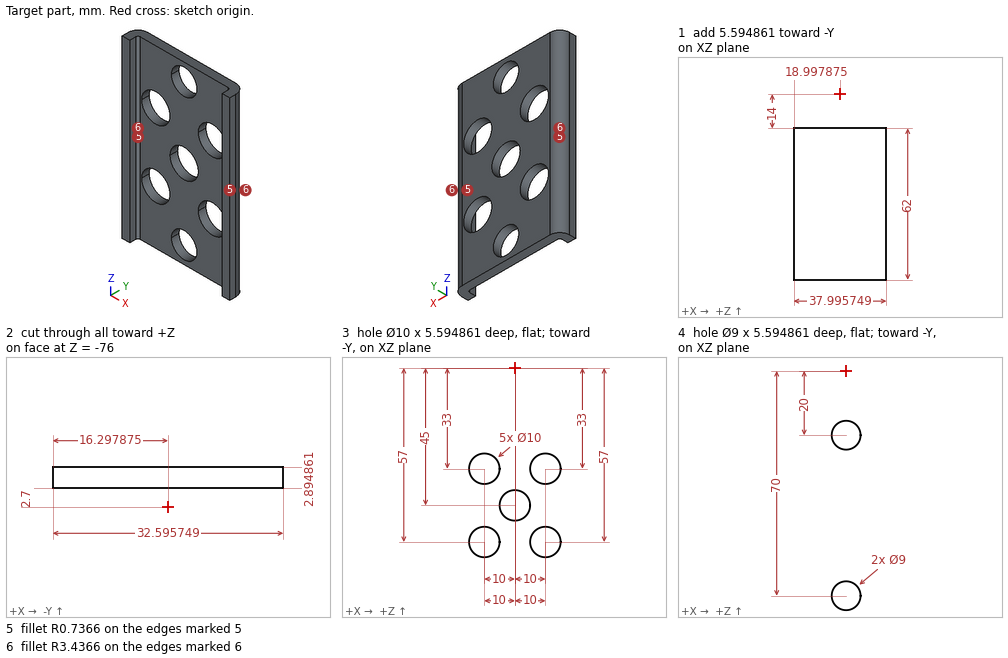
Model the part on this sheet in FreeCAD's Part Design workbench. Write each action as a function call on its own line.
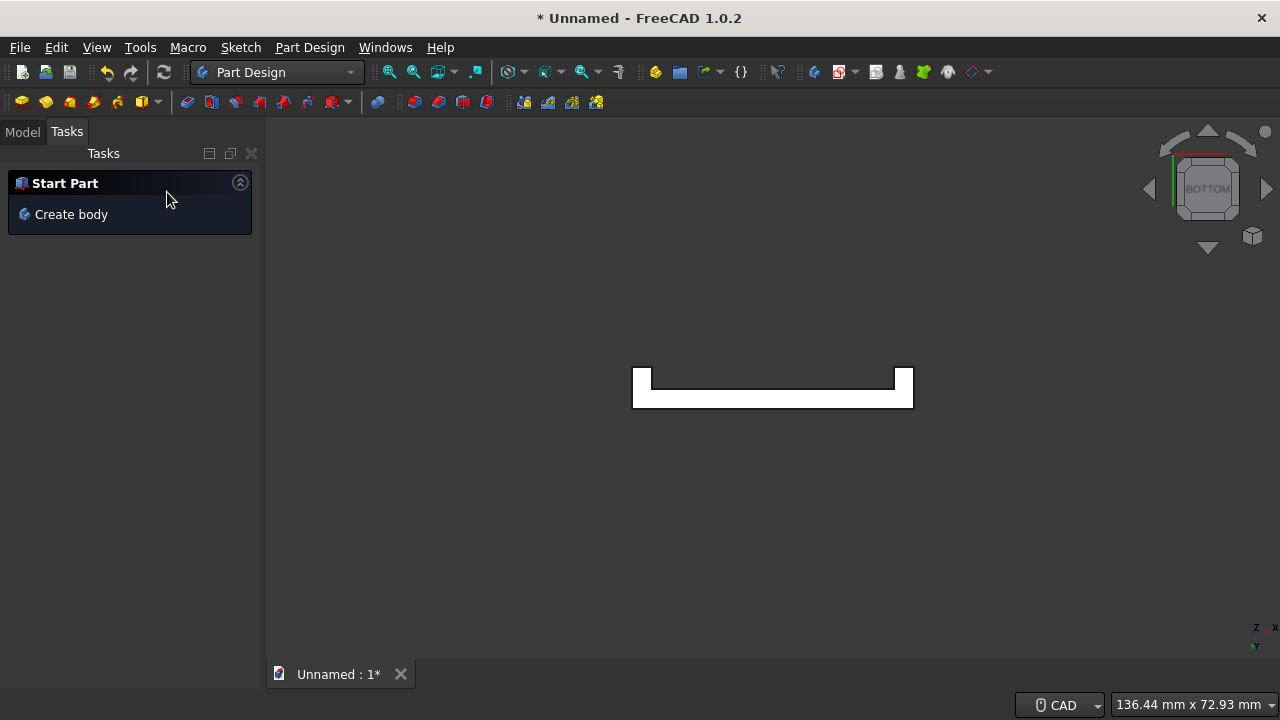
click(390, 72)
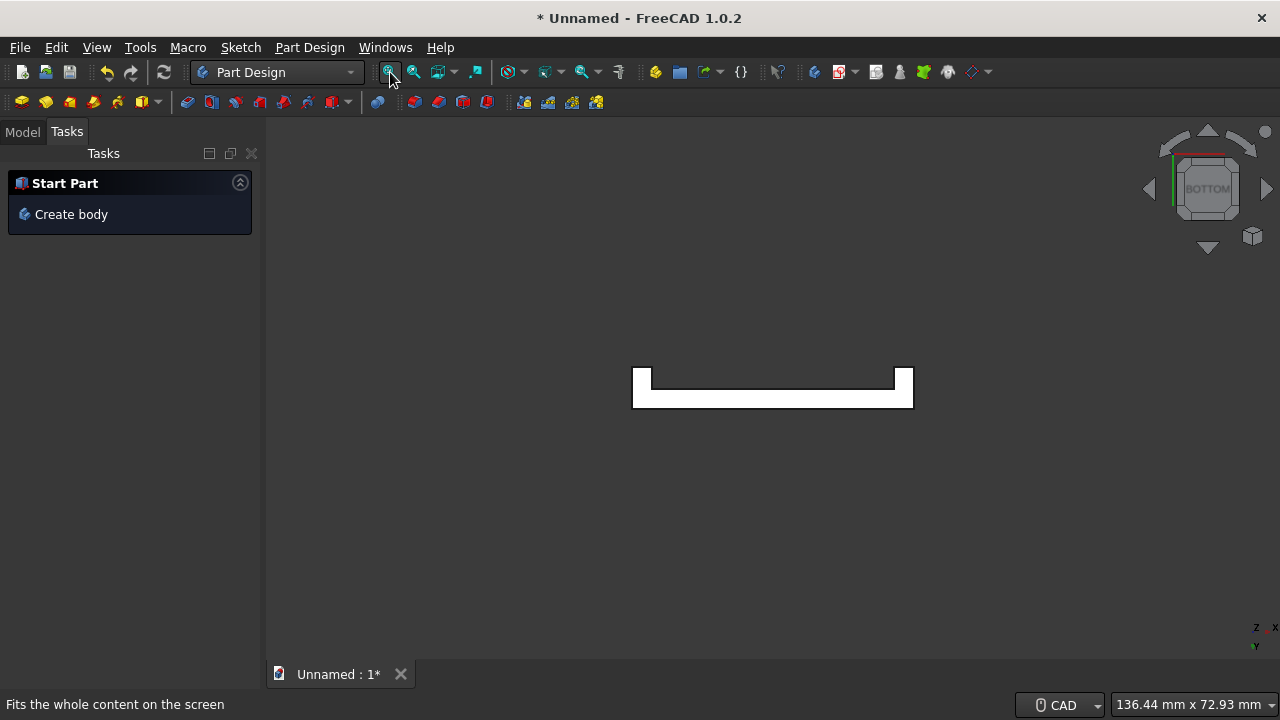
key(0)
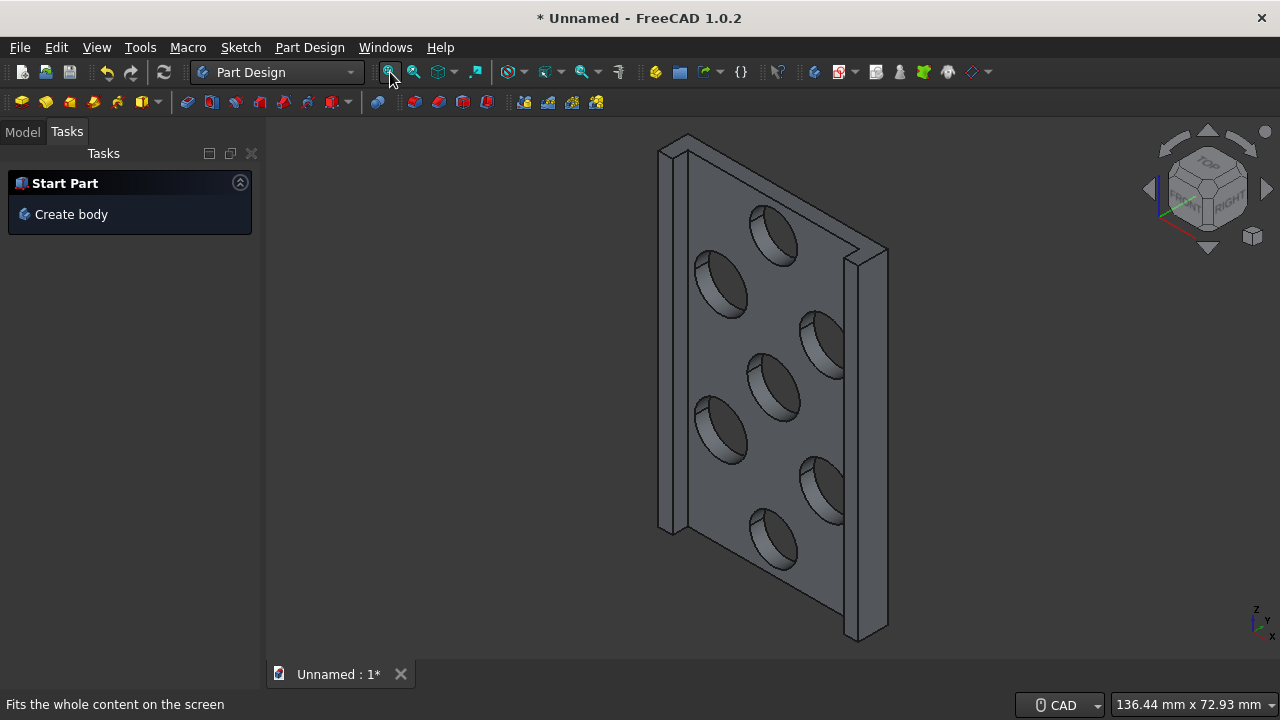
key(2)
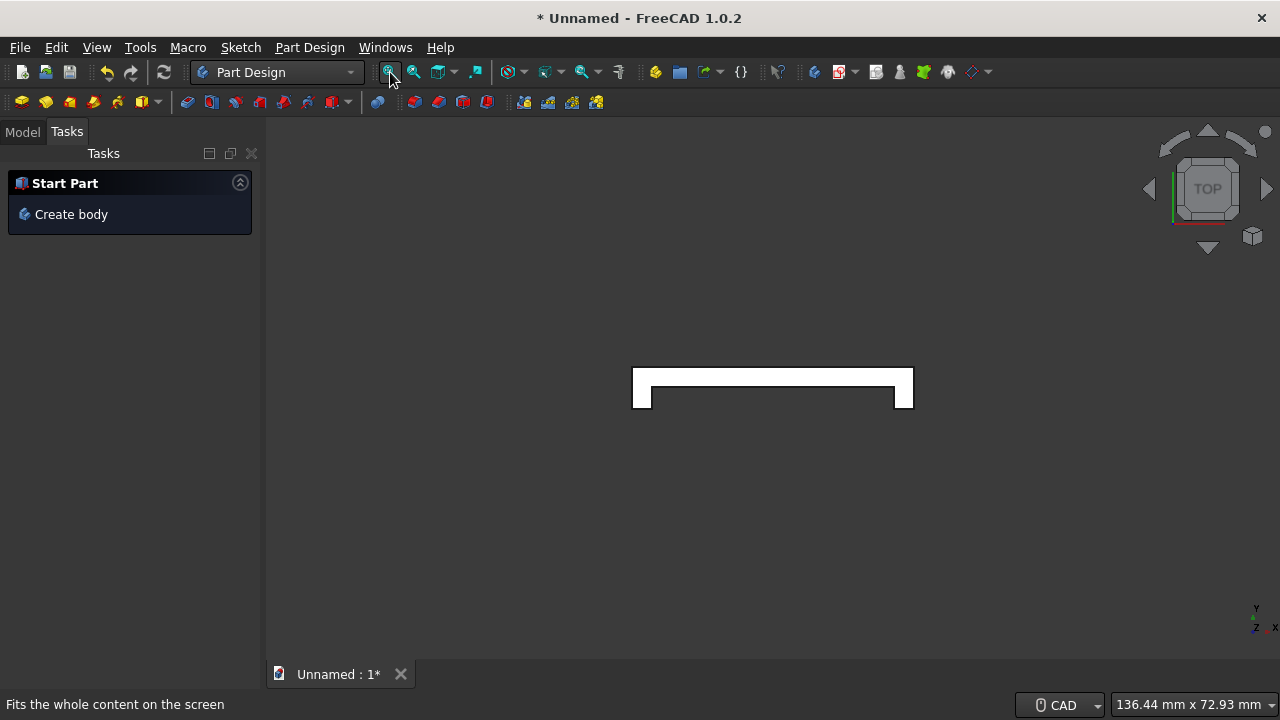
key(v)
key(f)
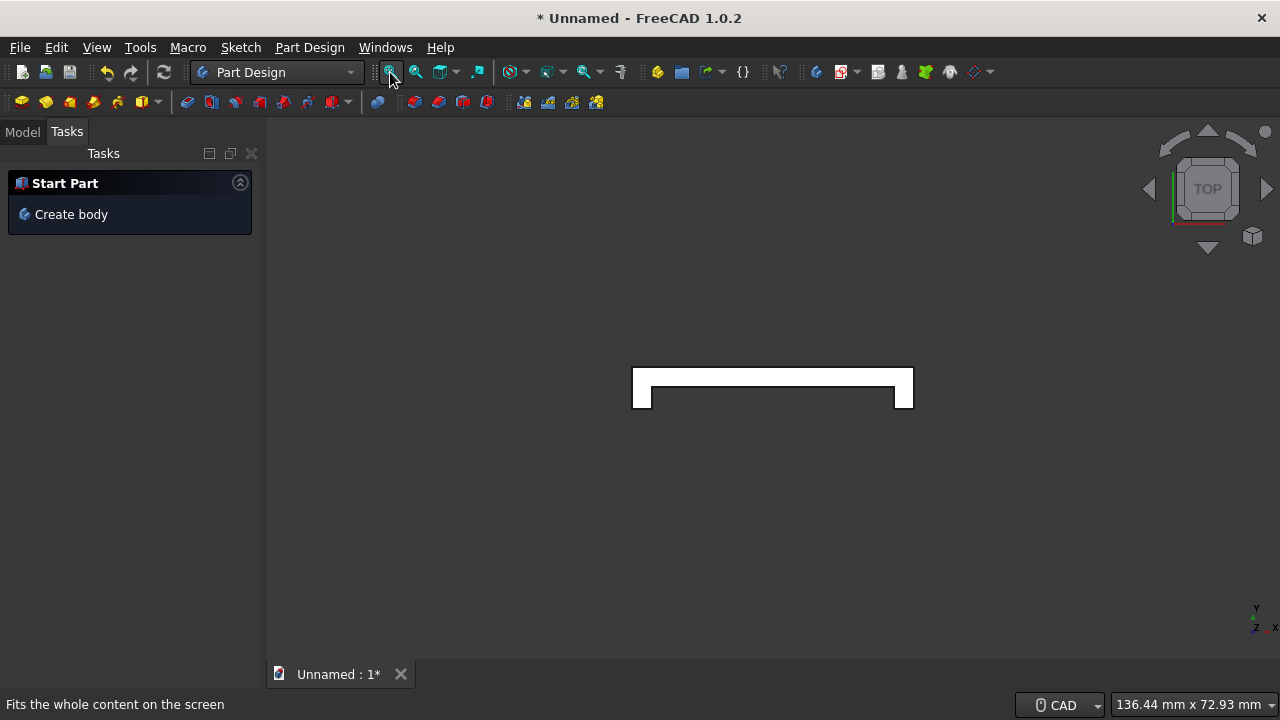
key(1)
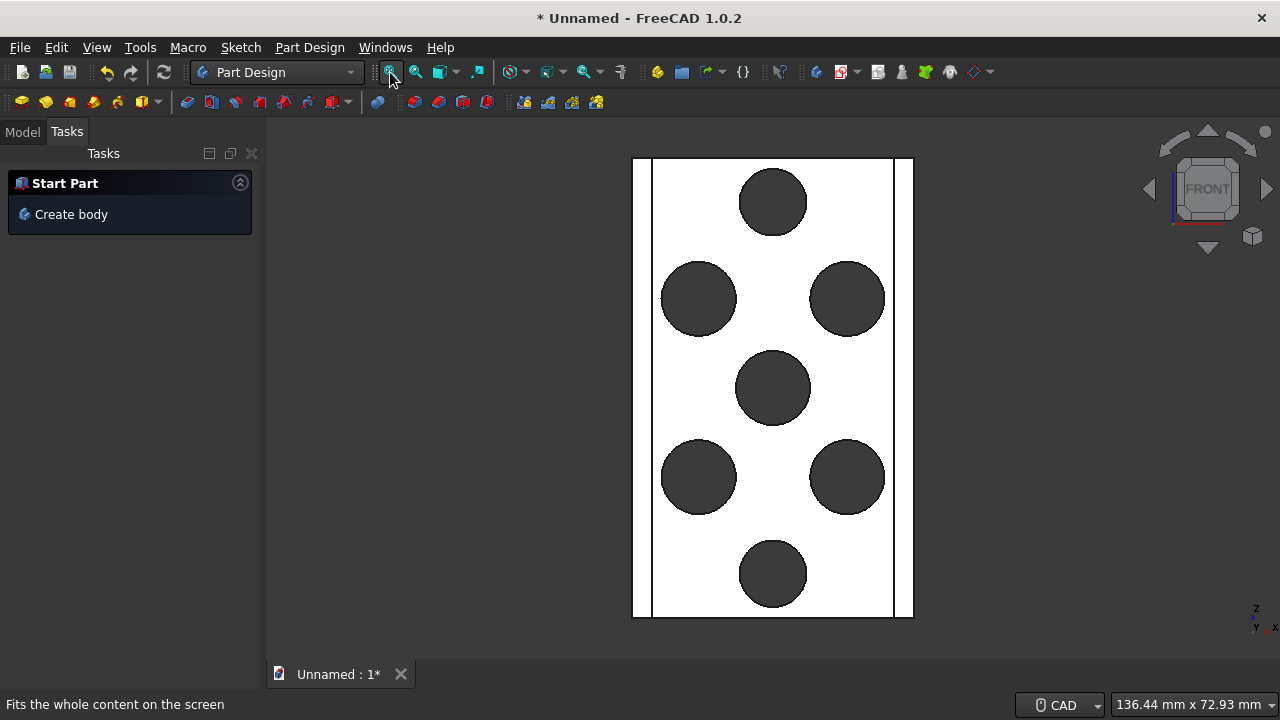
key(3)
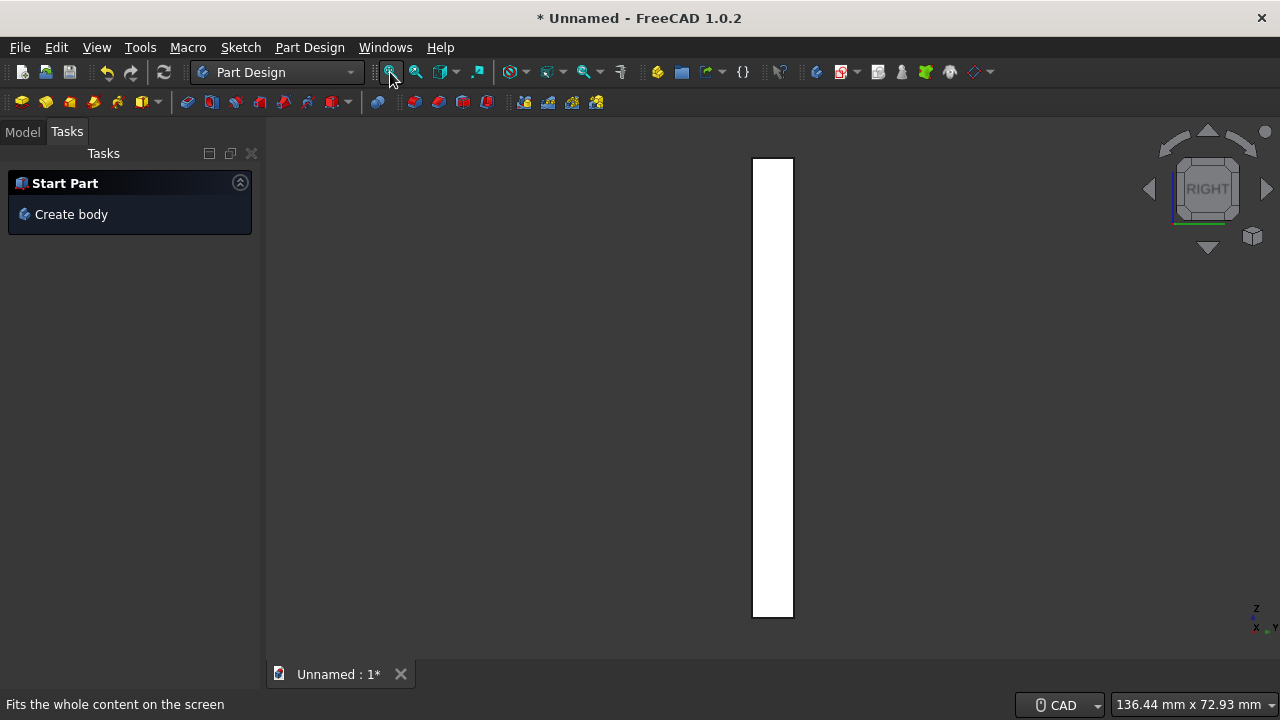
key(5)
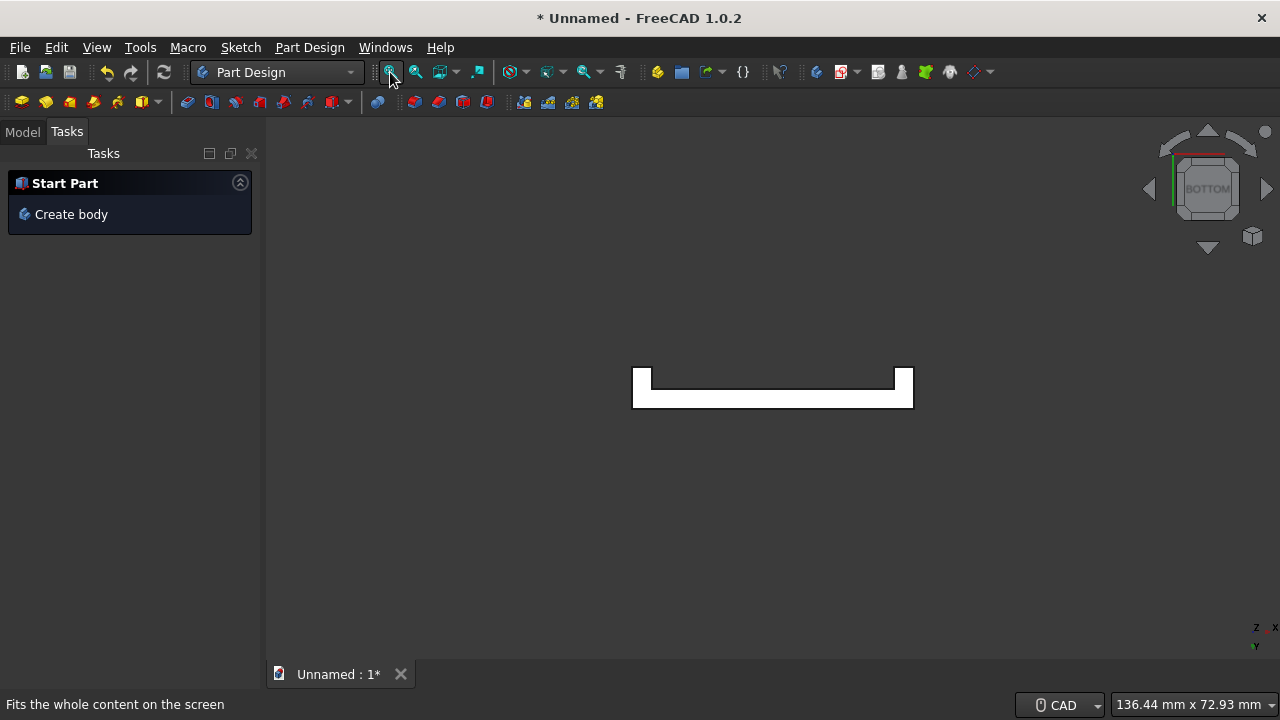
key(v)
key(f)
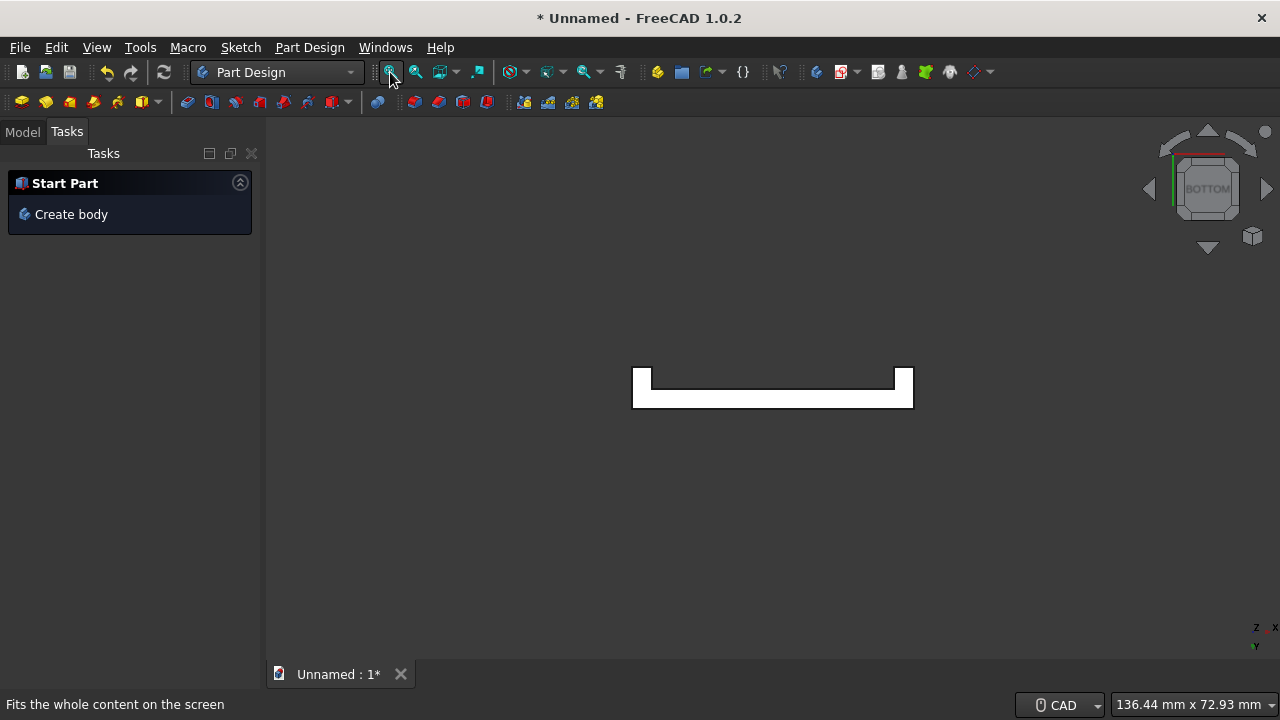
key(4)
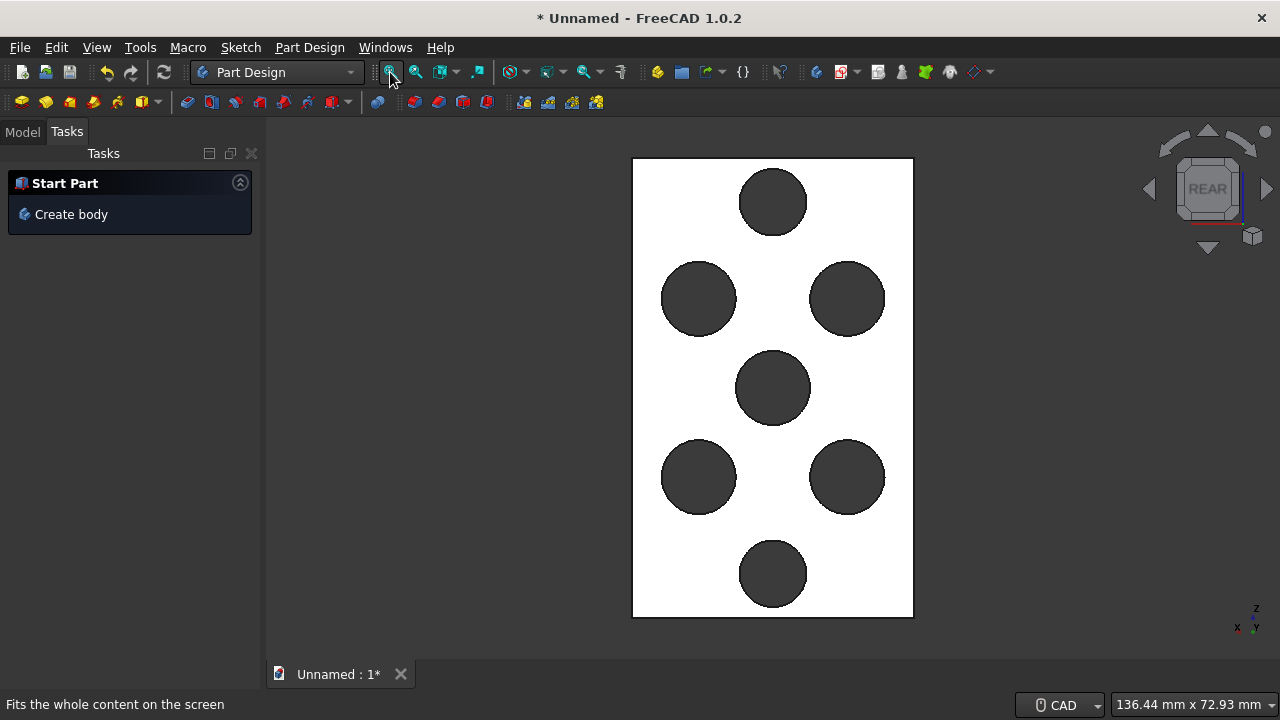
key(6)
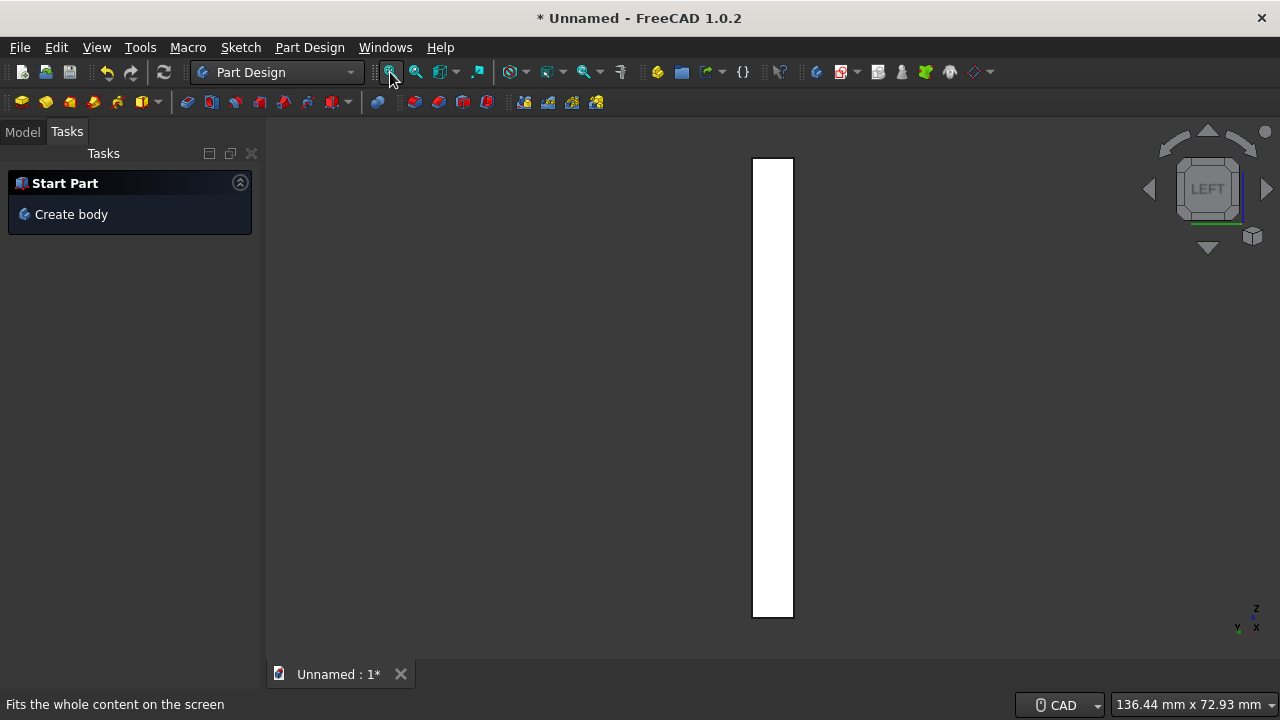
key(v)
key(3)